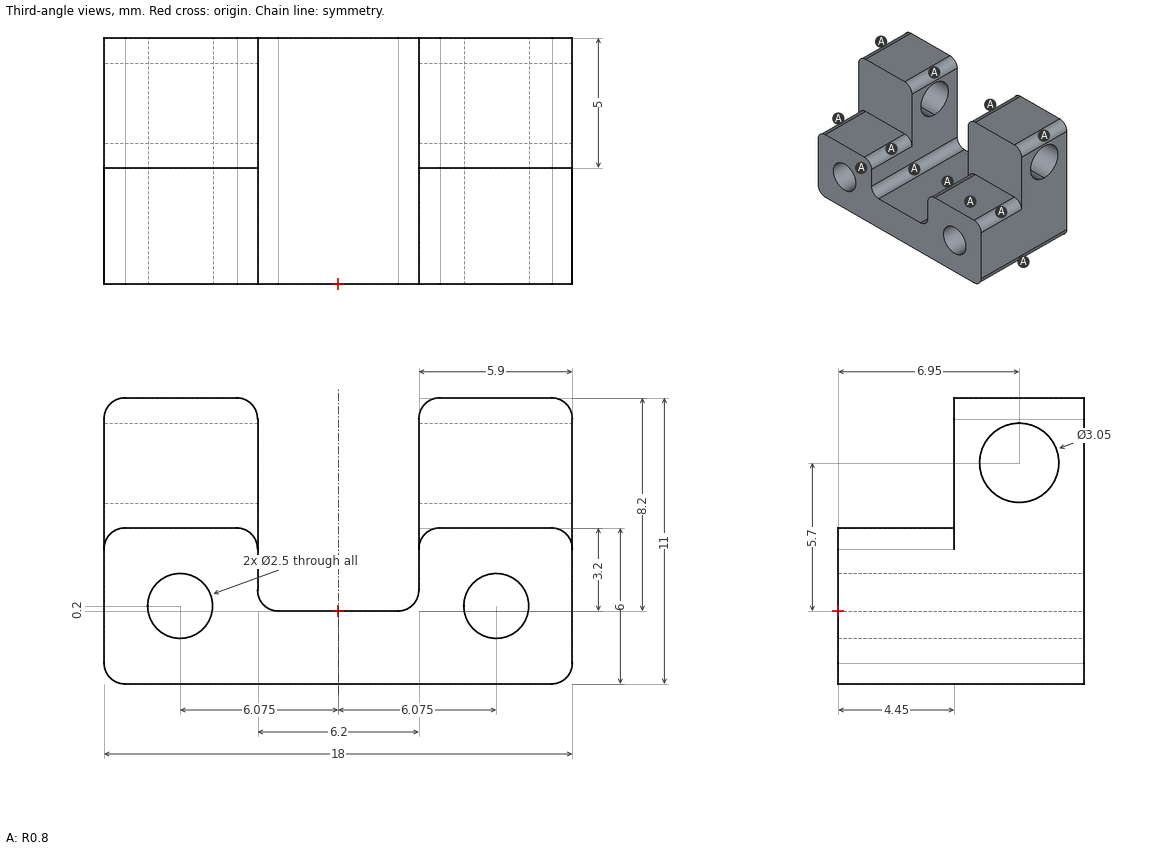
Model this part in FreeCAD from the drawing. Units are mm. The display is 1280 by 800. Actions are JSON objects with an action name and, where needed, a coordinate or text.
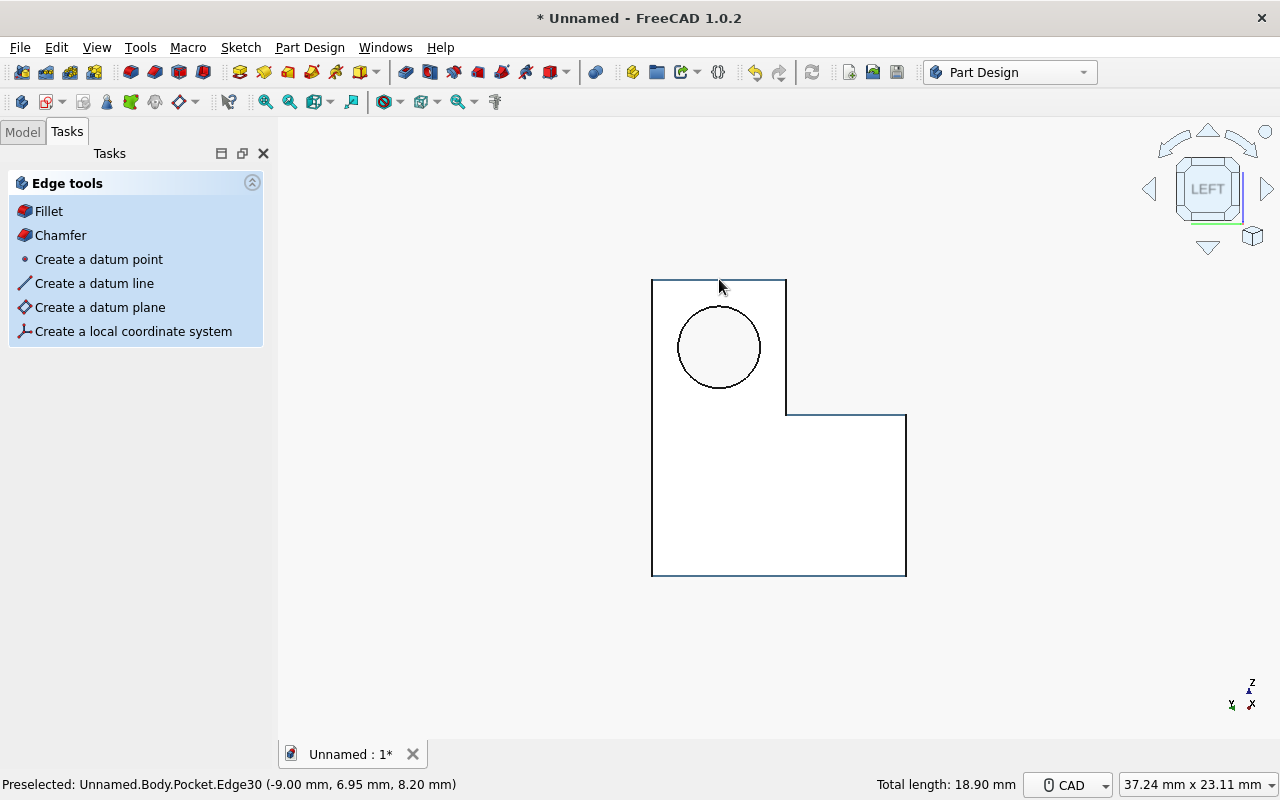
{"action": "key", "text": "0"}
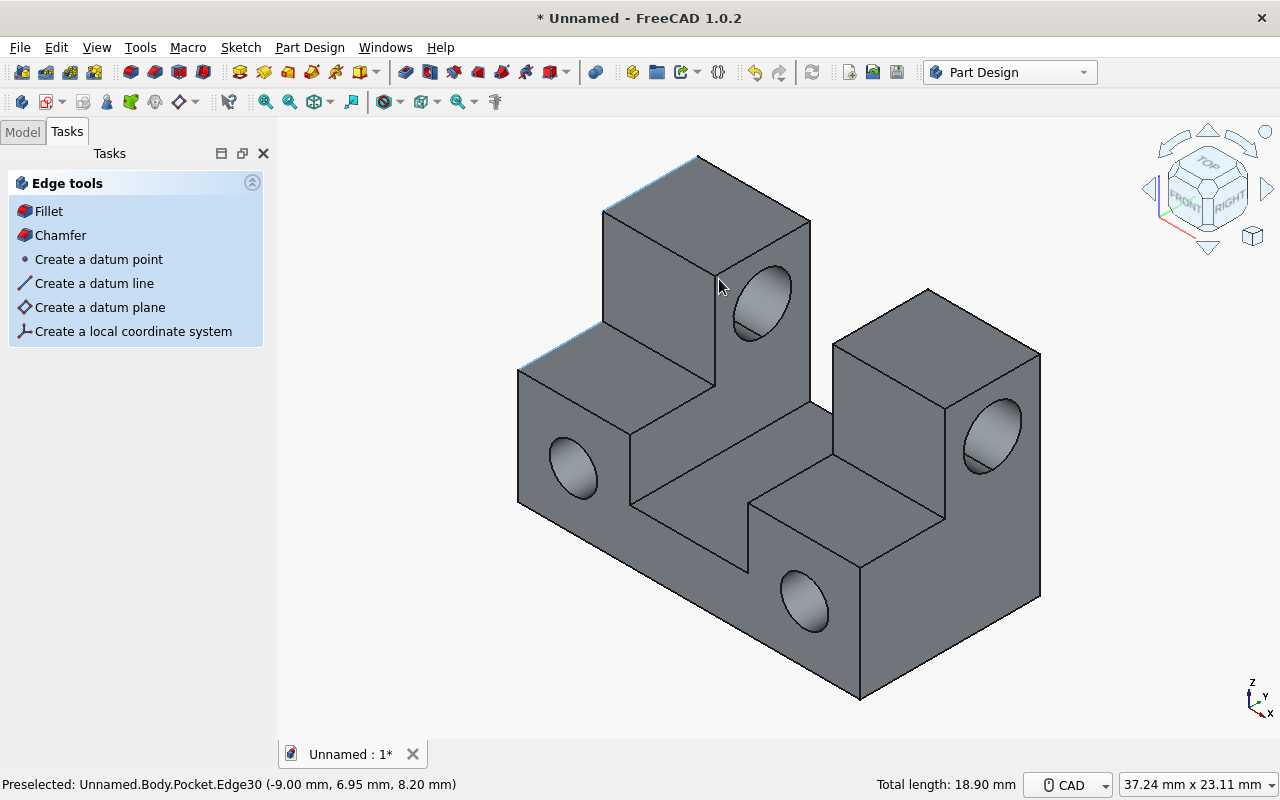
{"action": "left_click", "coordinate": [903, 542], "text": "ctrl"}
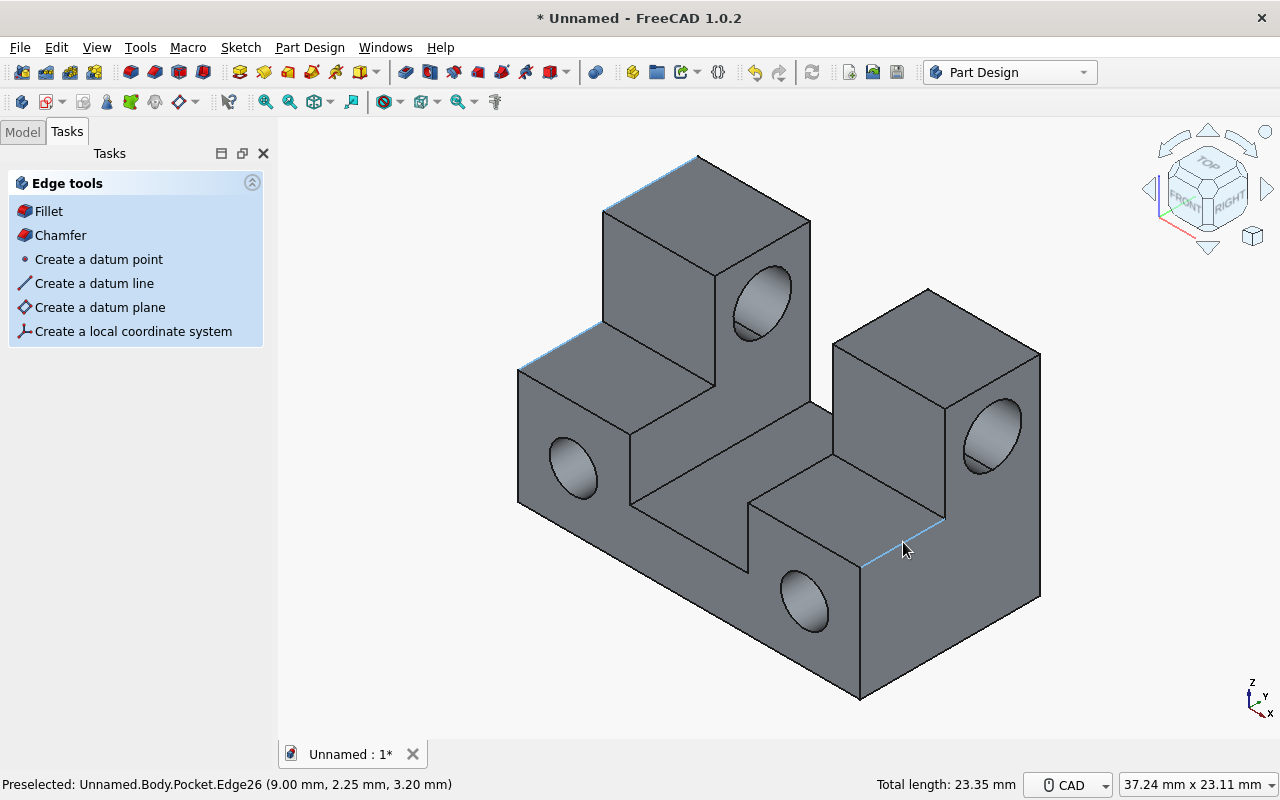
{"action": "left_click", "coordinate": [672, 409], "text": "ctrl"}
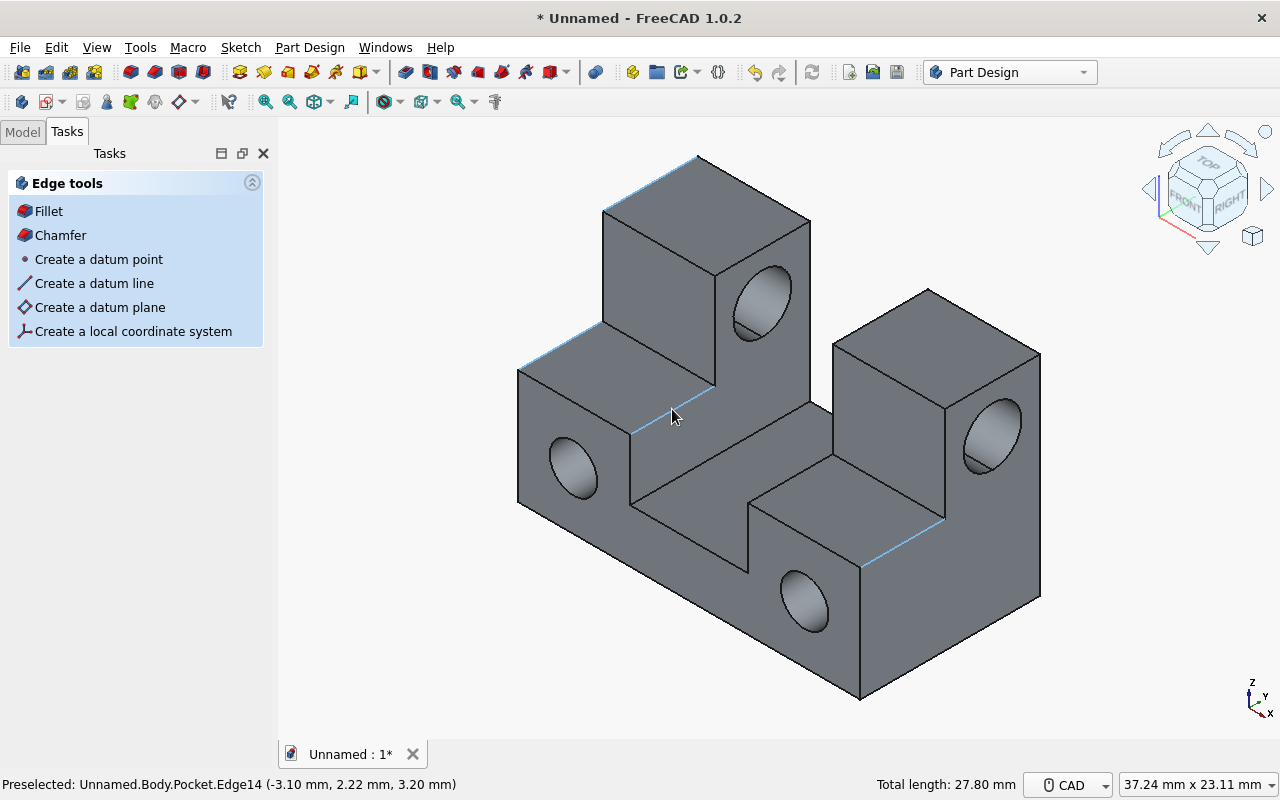
{"action": "left_click", "coordinate": [762, 248], "text": "ctrl"}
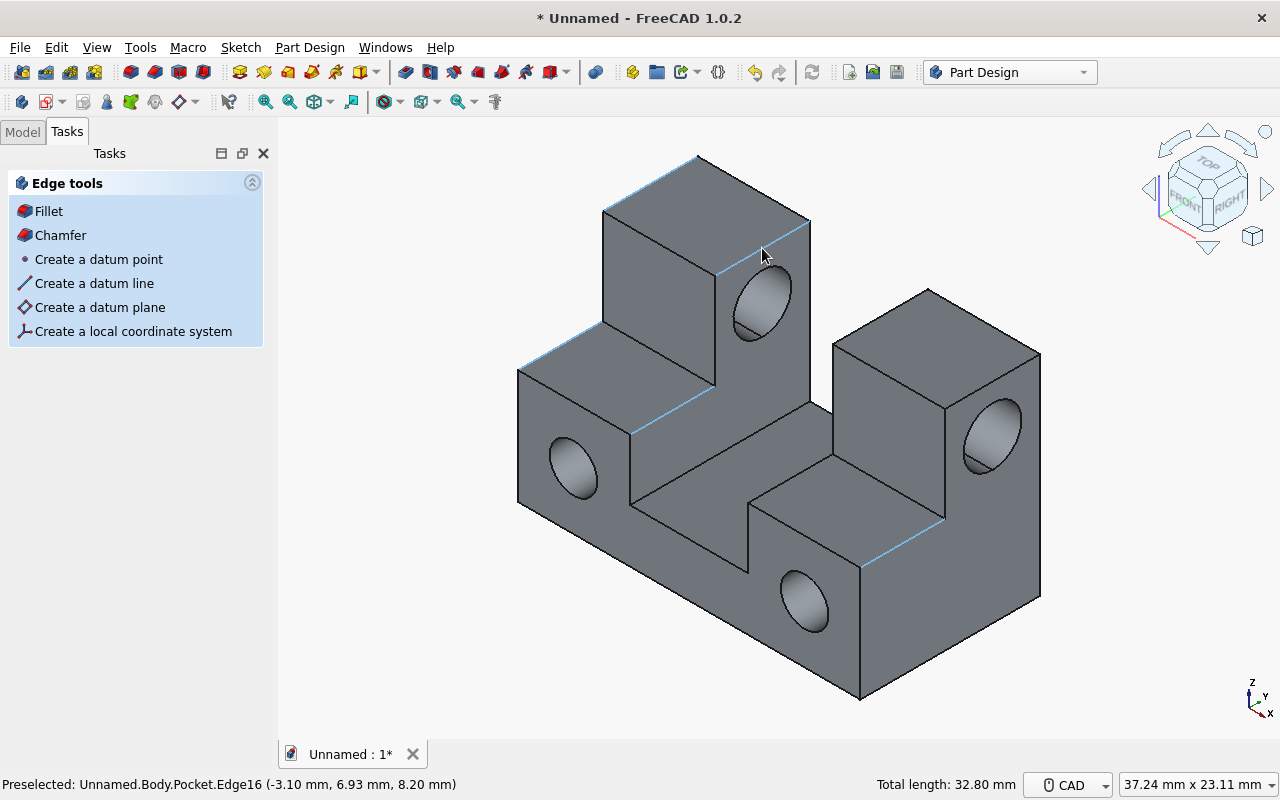
{"action": "left_click", "coordinate": [993, 381], "text": "ctrl"}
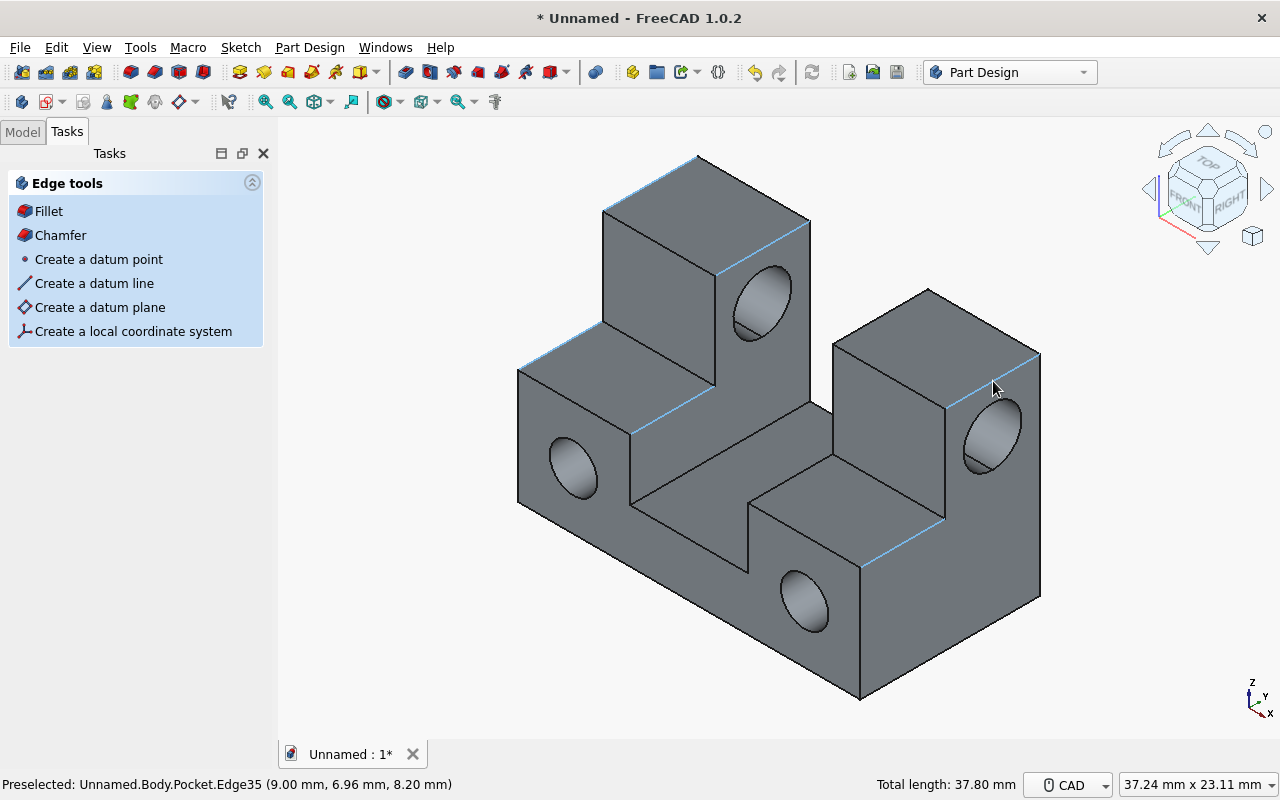
{"action": "key", "text": "2"}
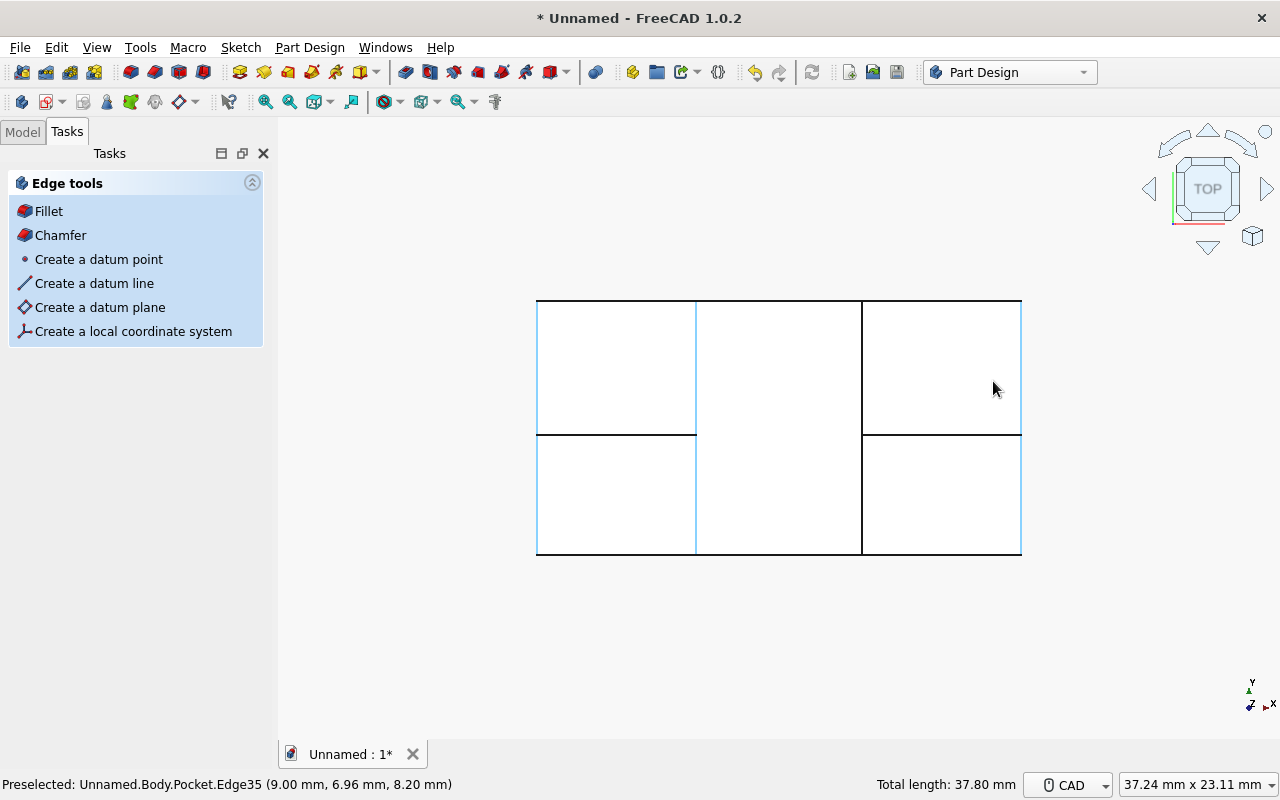
{"action": "left_click", "coordinate": [862, 494], "text": "ctrl"}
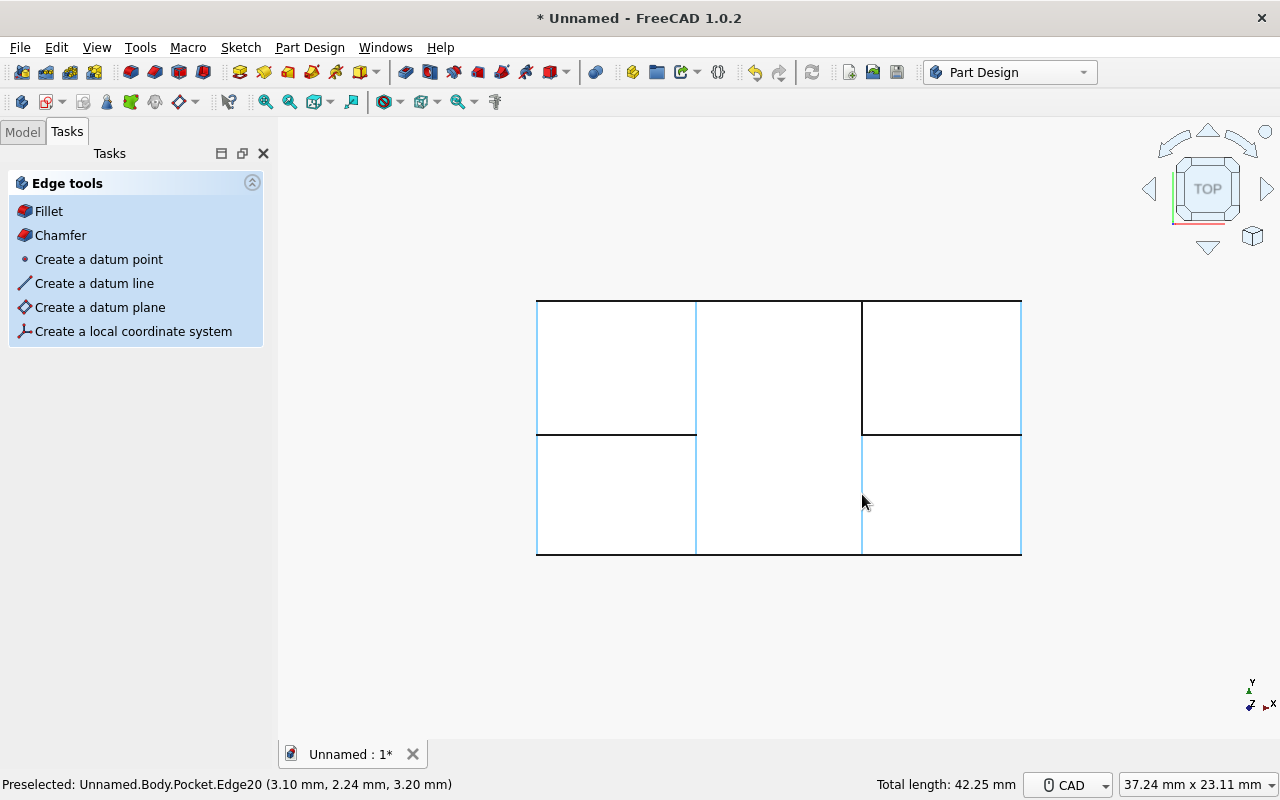
{"action": "left_click", "coordinate": [862, 367], "text": "ctrl"}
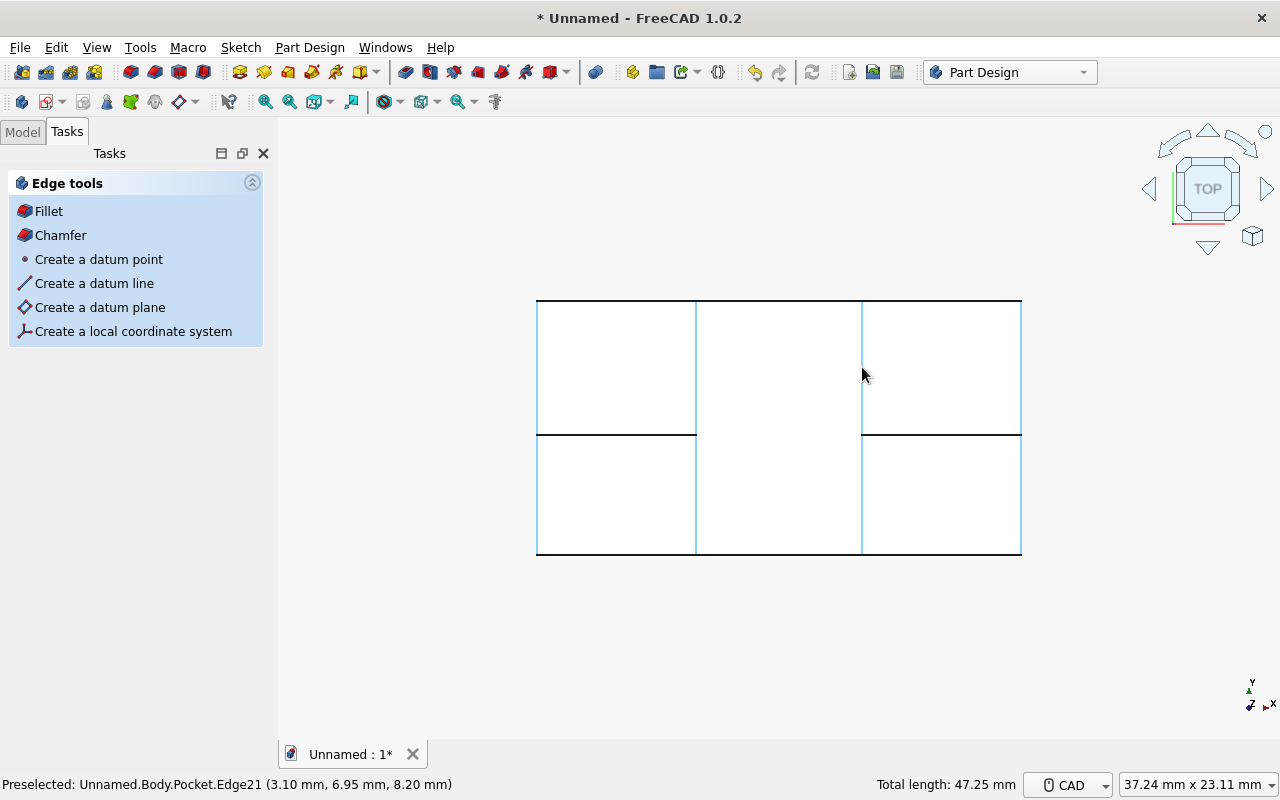
{"action": "key", "text": "1"}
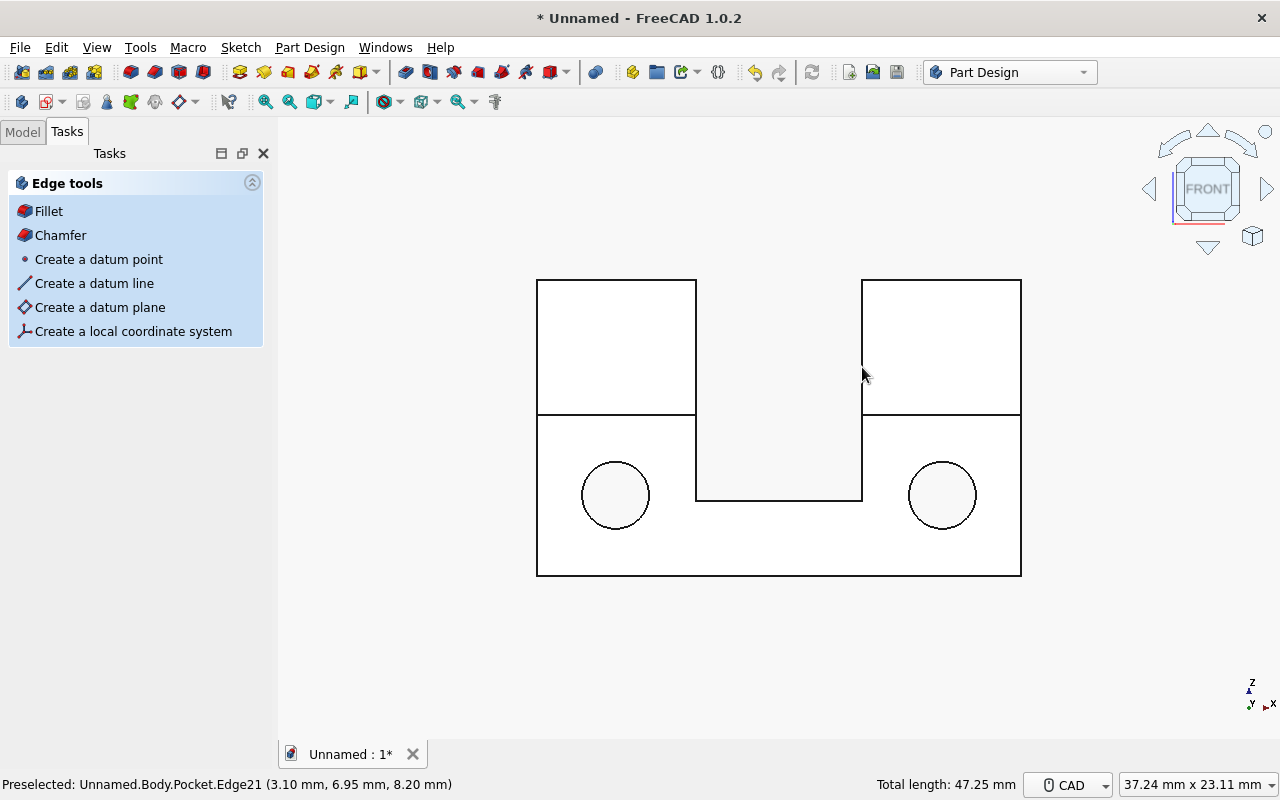
{"action": "key", "text": "3"}